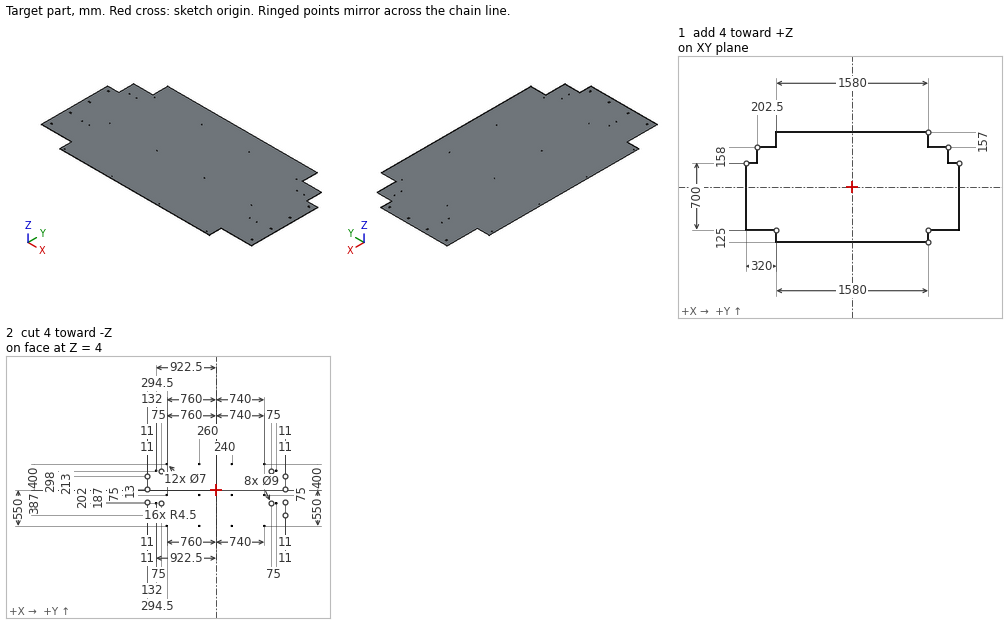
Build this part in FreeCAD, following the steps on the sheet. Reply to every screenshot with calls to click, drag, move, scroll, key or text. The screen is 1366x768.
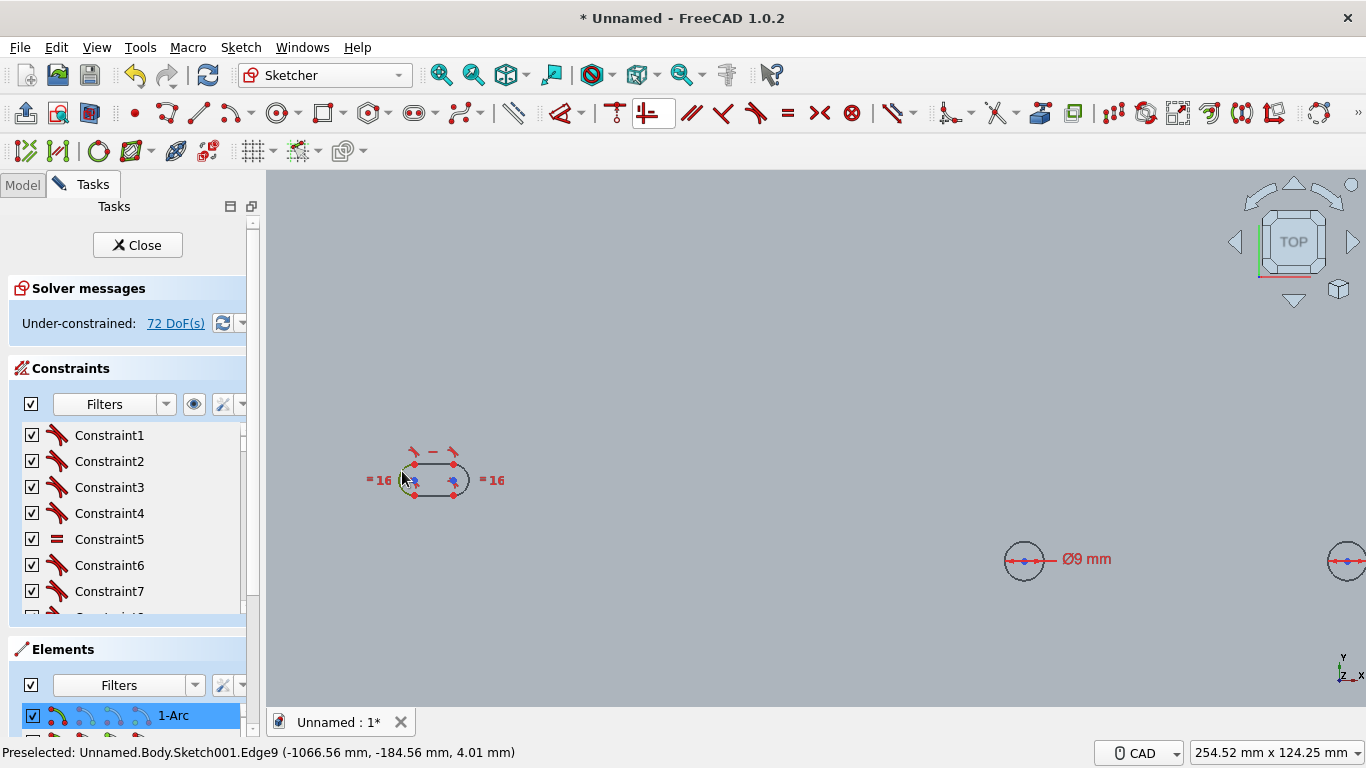
scroll(405, 474, down, 13)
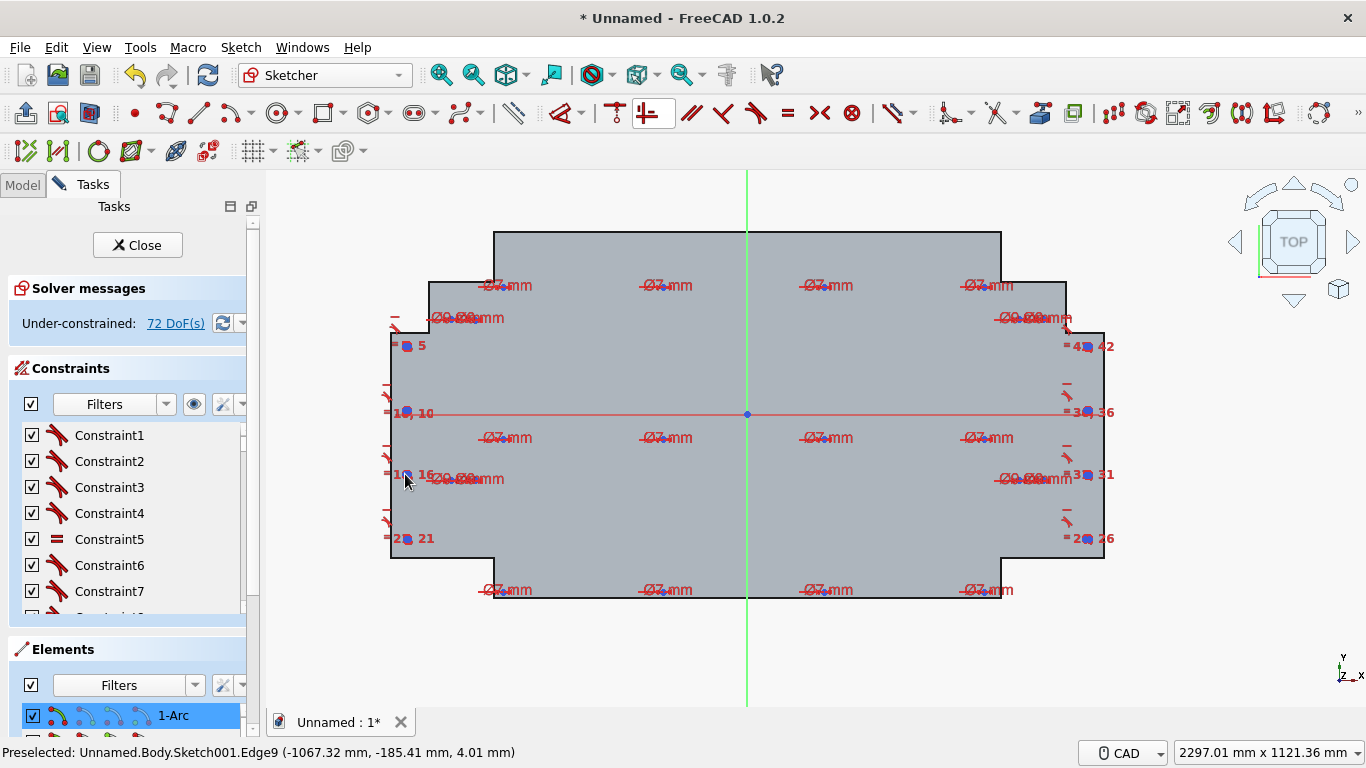
scroll(404, 538, up, 10)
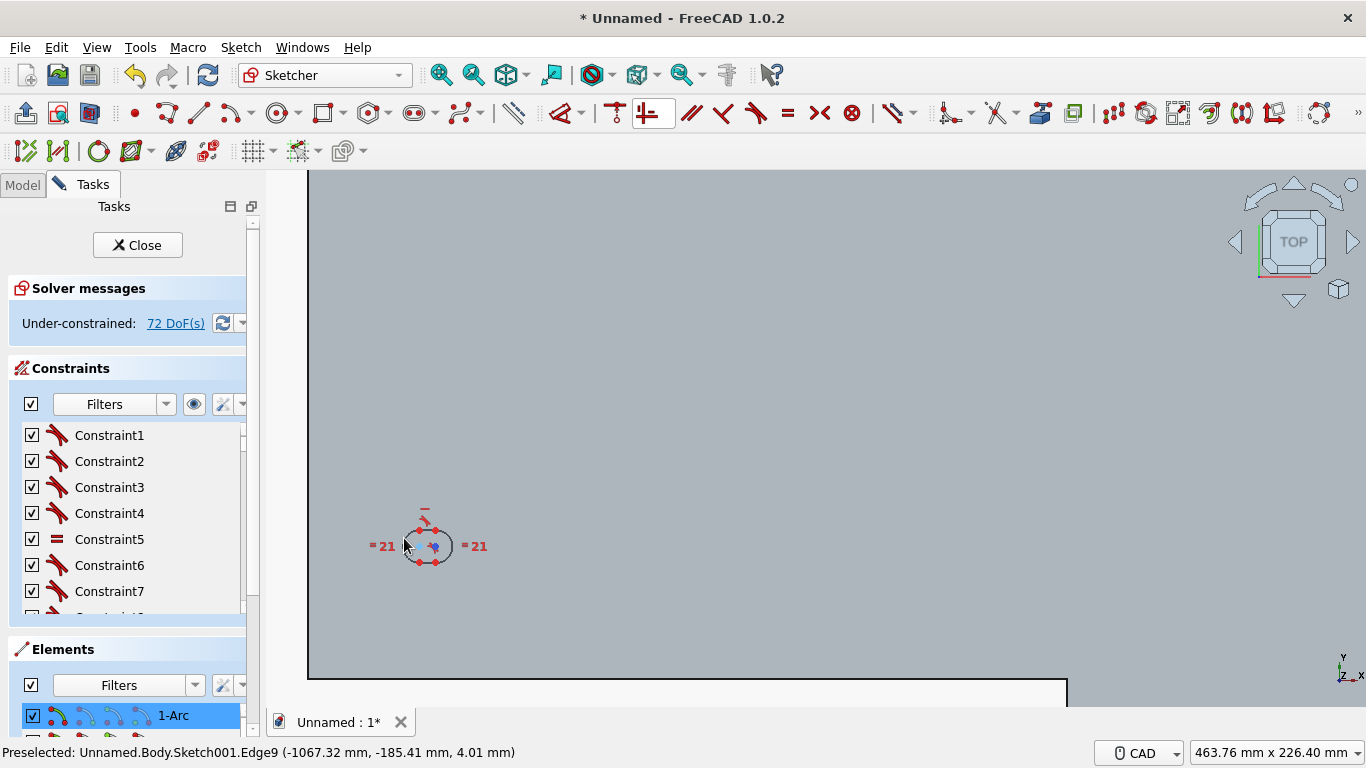
click(406, 537)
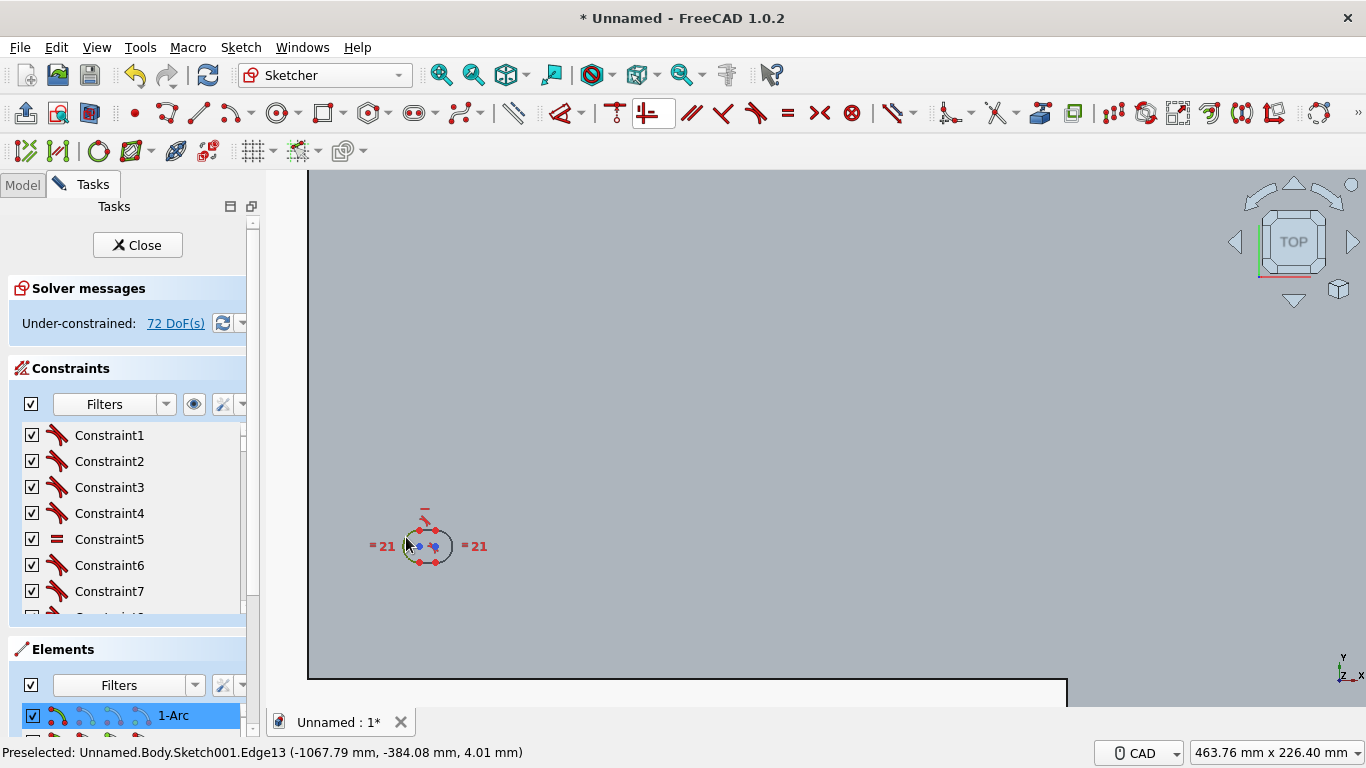
scroll(404, 538, down, 10)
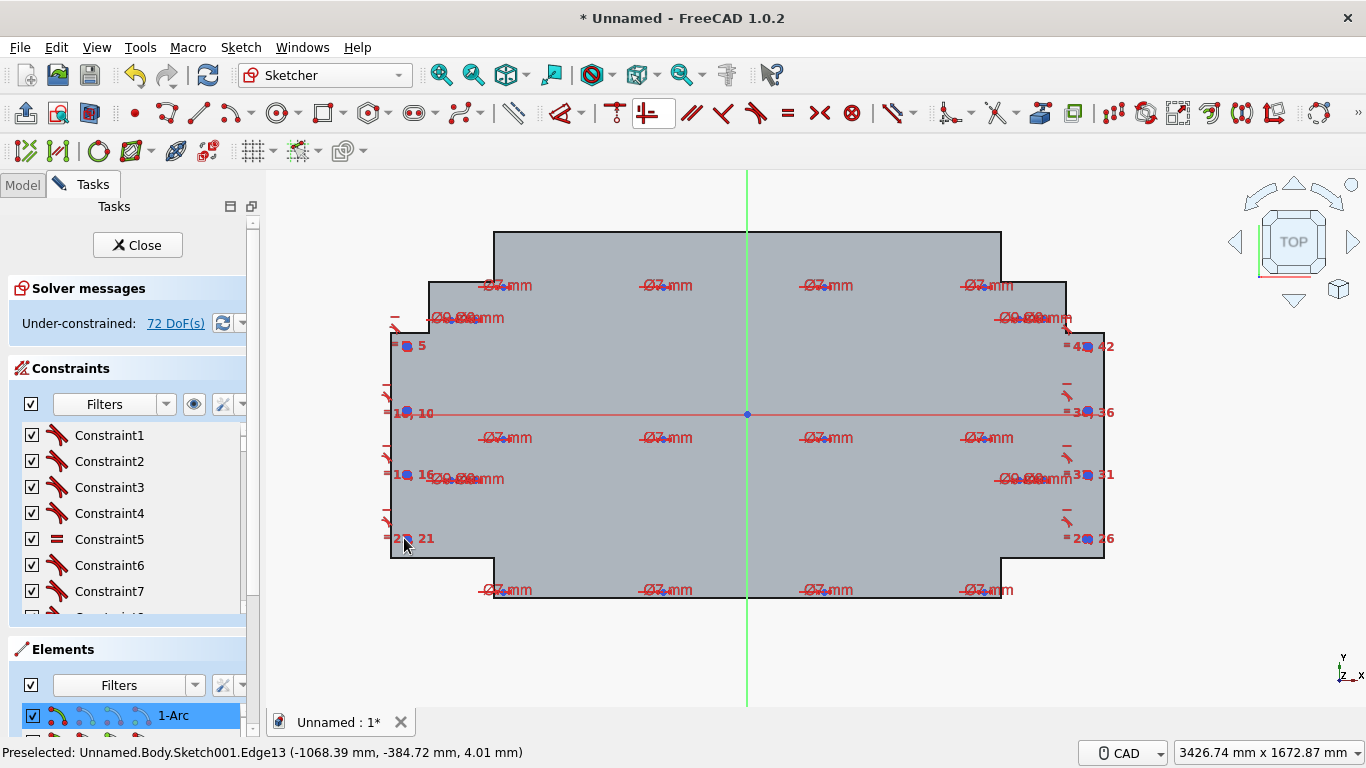
scroll(1084, 538, up, 11)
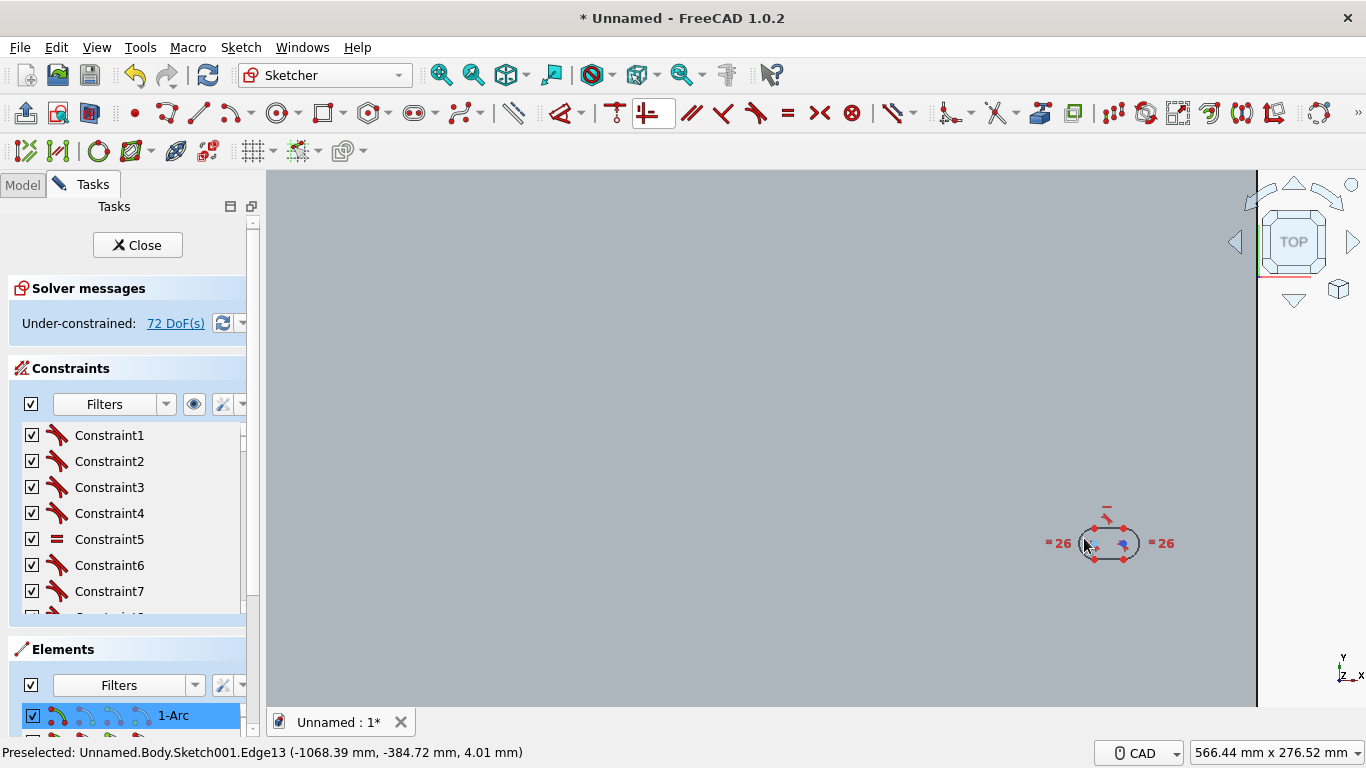
click(1082, 535)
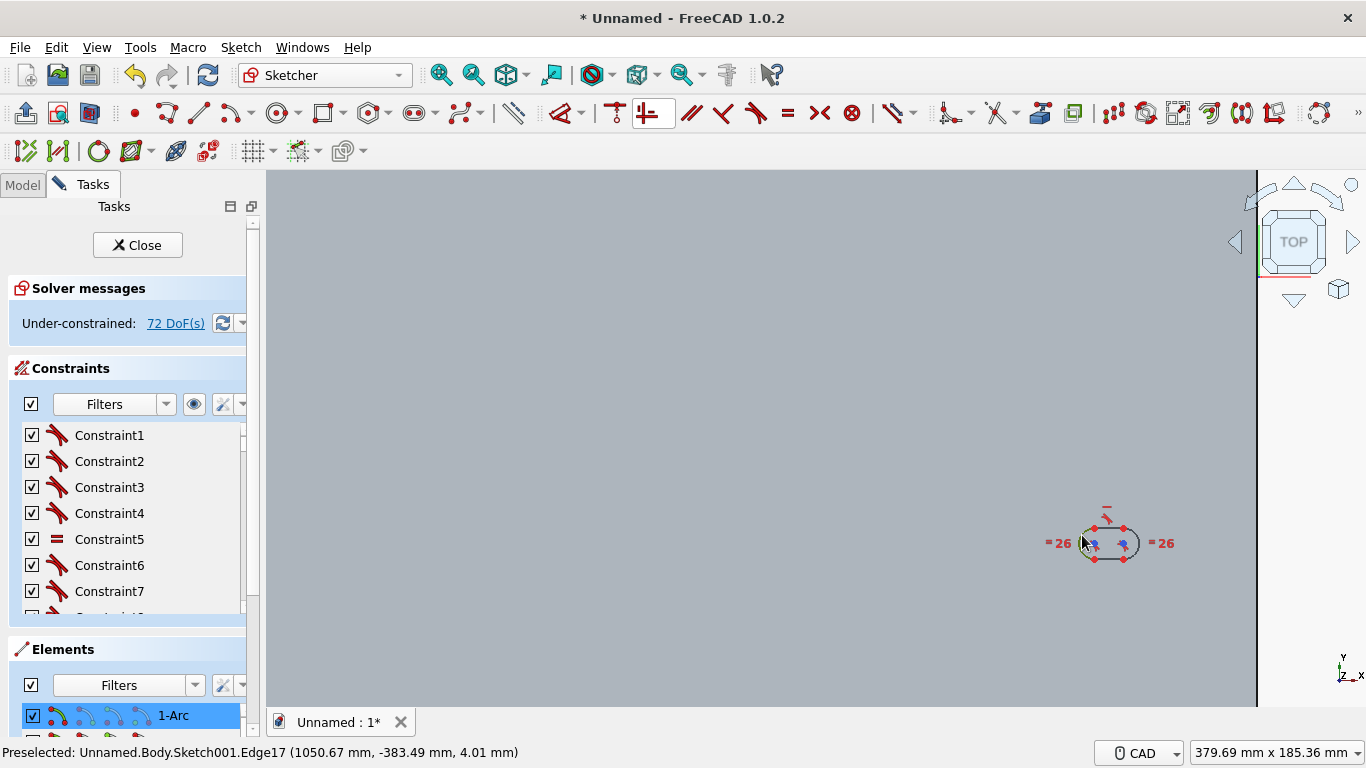
scroll(1085, 538, down, 11)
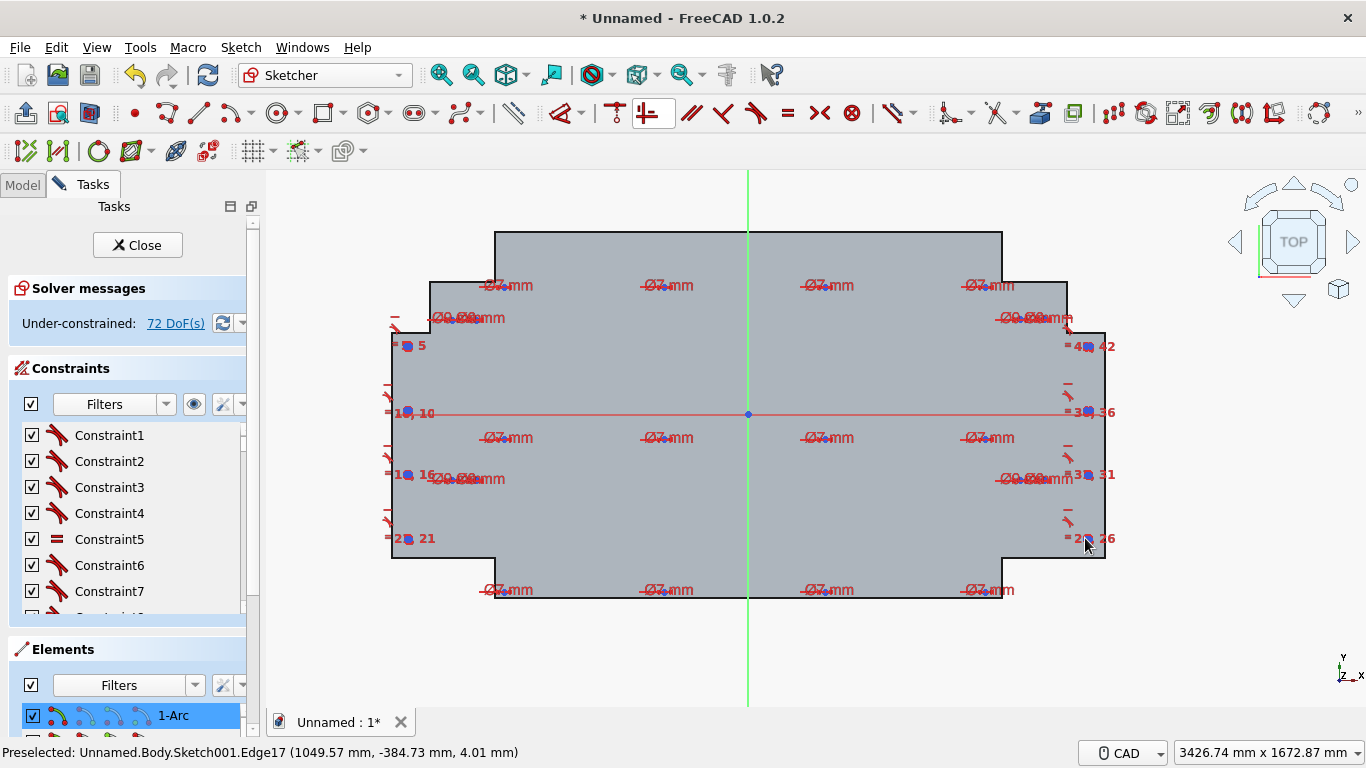
scroll(1086, 475, up, 12)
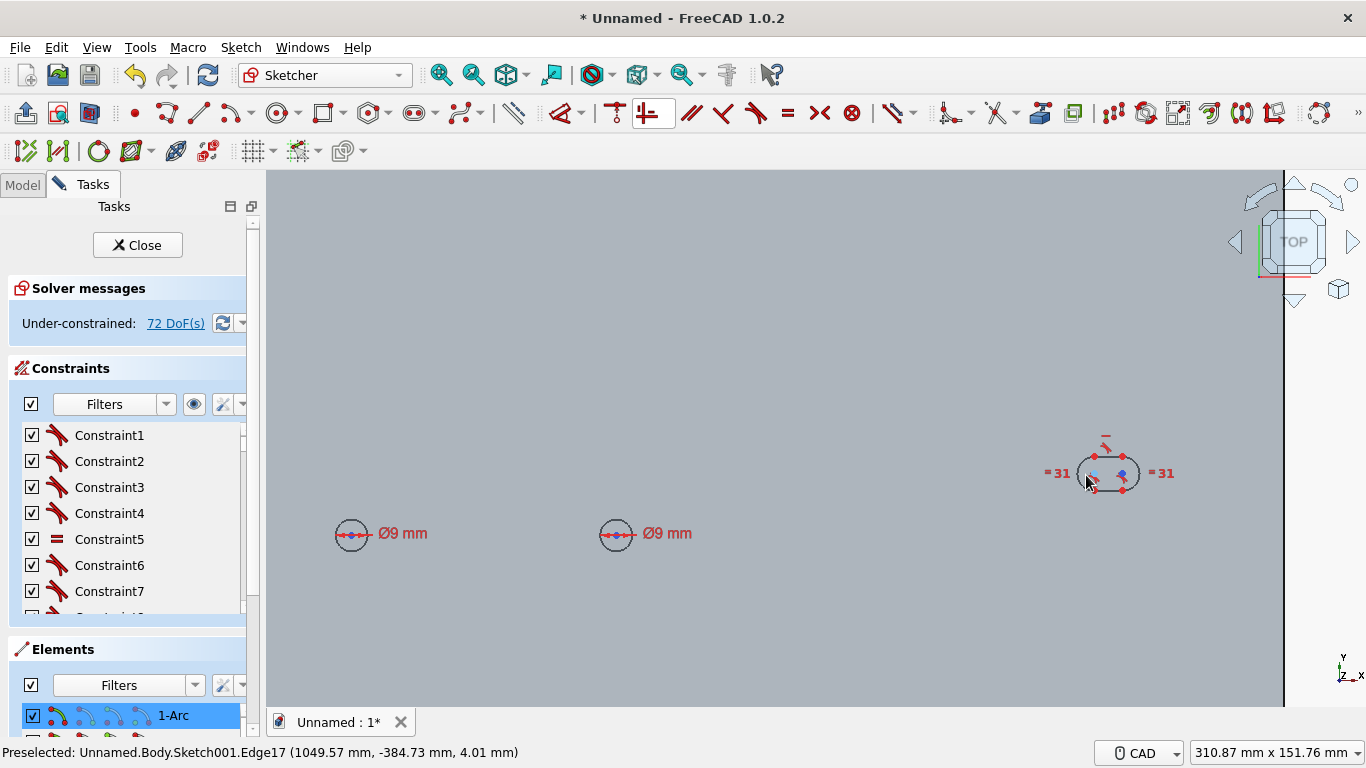
click(1081, 464)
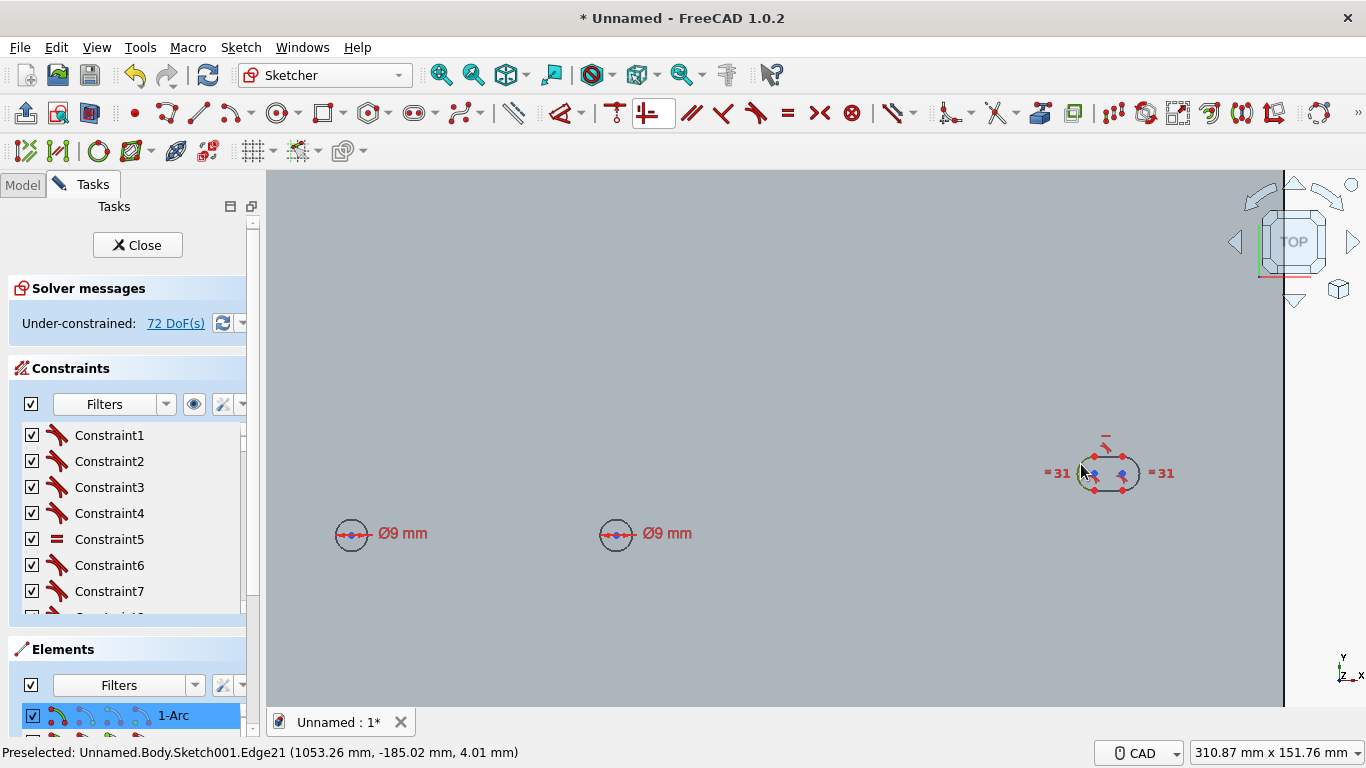
scroll(1086, 475, down, 12)